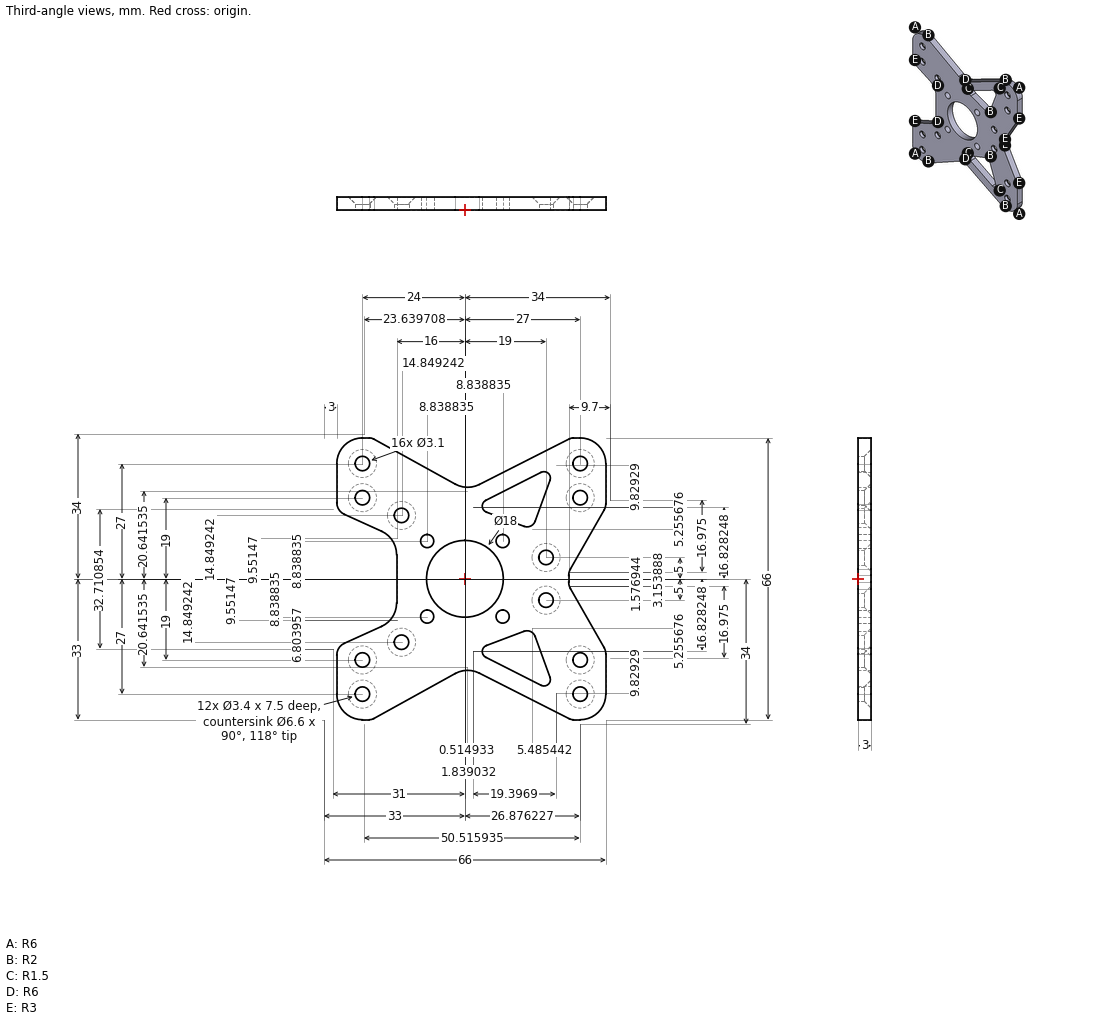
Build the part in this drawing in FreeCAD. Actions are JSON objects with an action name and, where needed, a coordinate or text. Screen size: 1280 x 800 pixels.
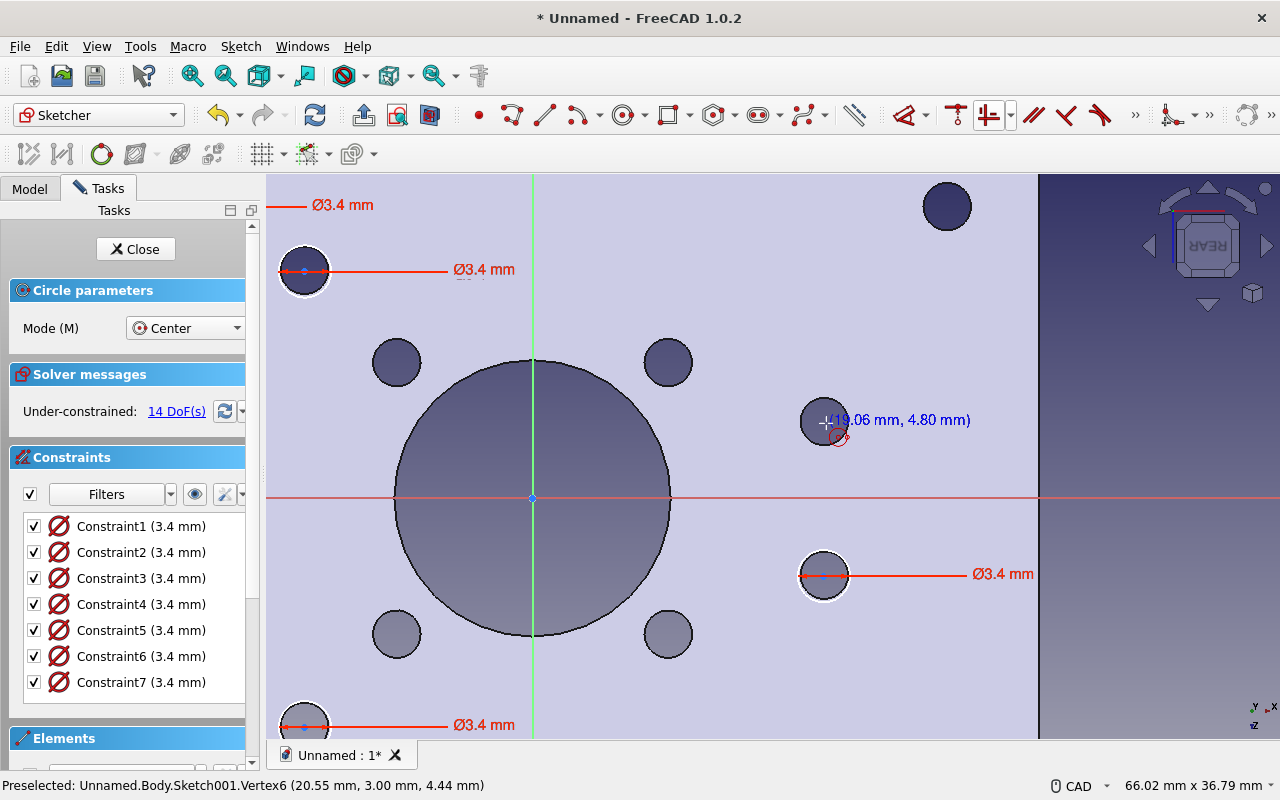
{"action": "left_click", "coordinate": [824, 422]}
{"action": "mouse_move", "coordinate": [843, 403]}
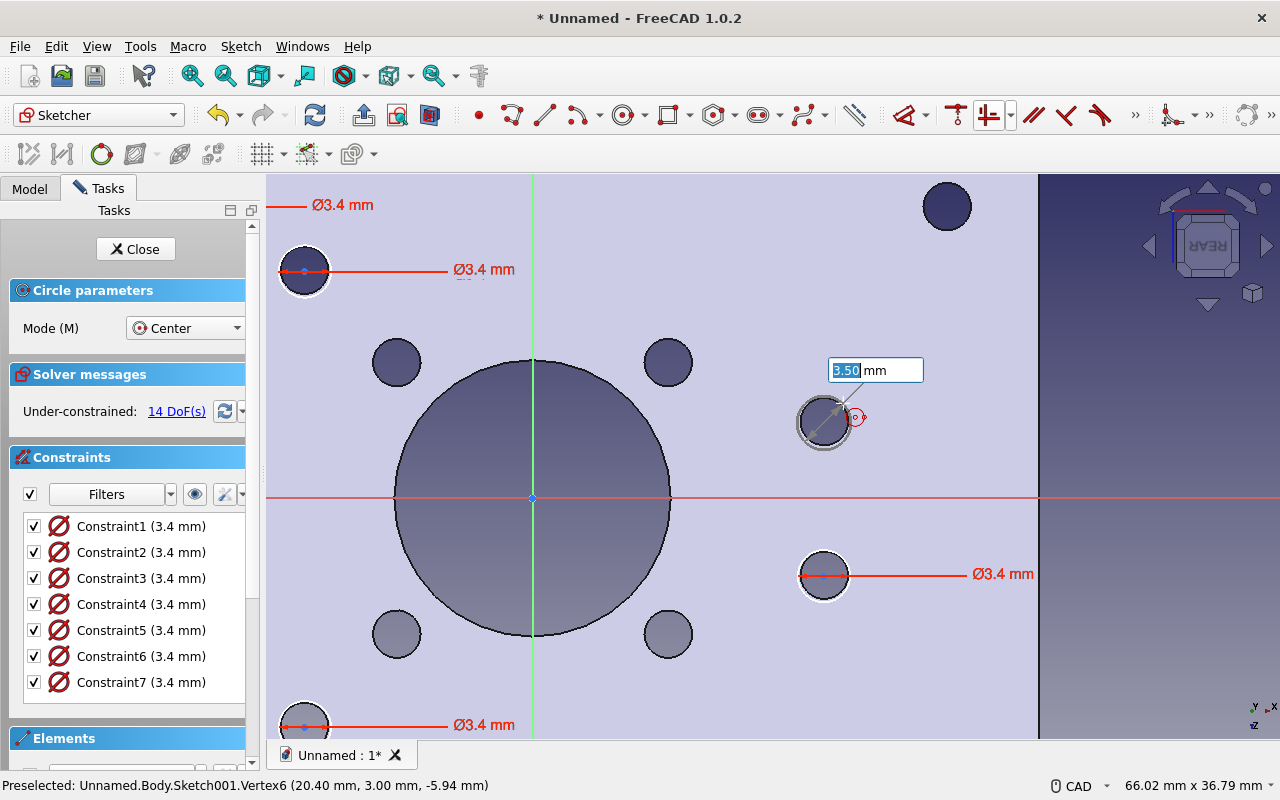
{"action": "type", "text": "3.4"}
{"action": "key", "text": "Return"}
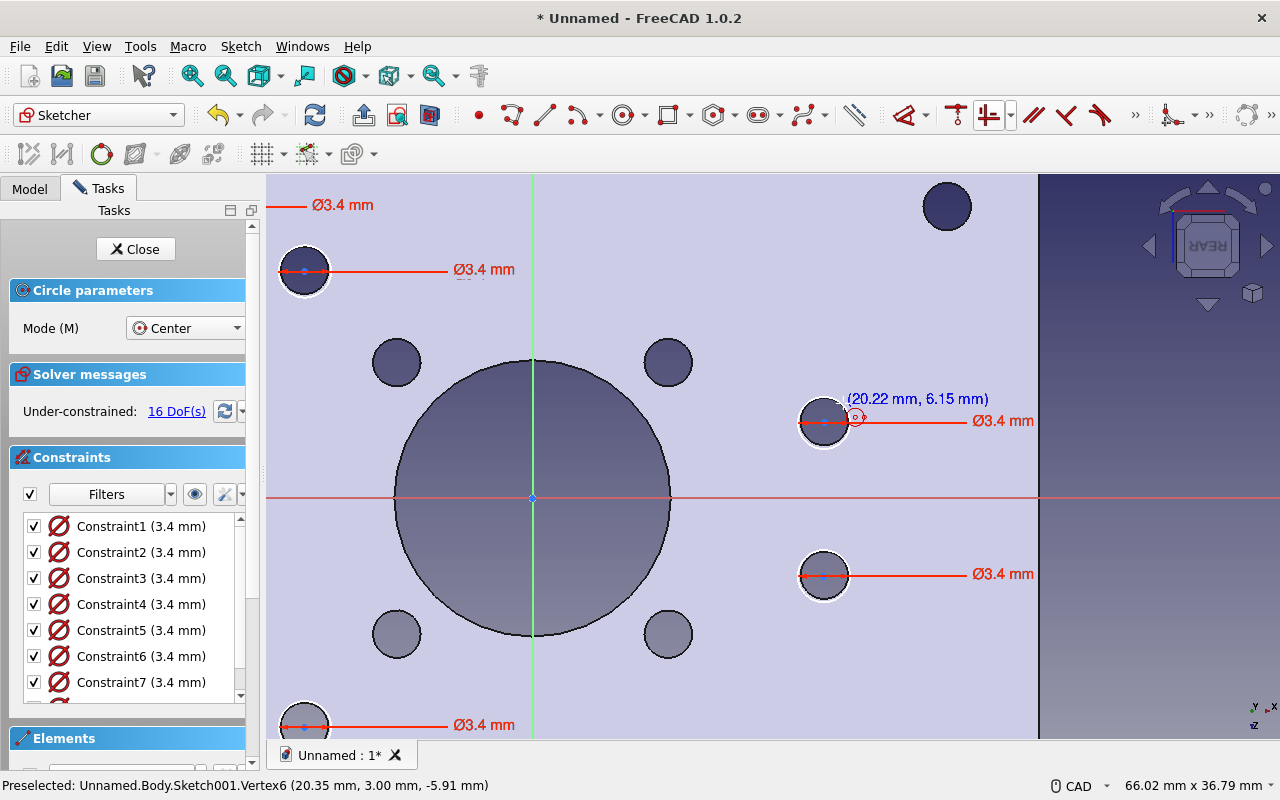
{"action": "left_click", "coordinate": [947, 207]}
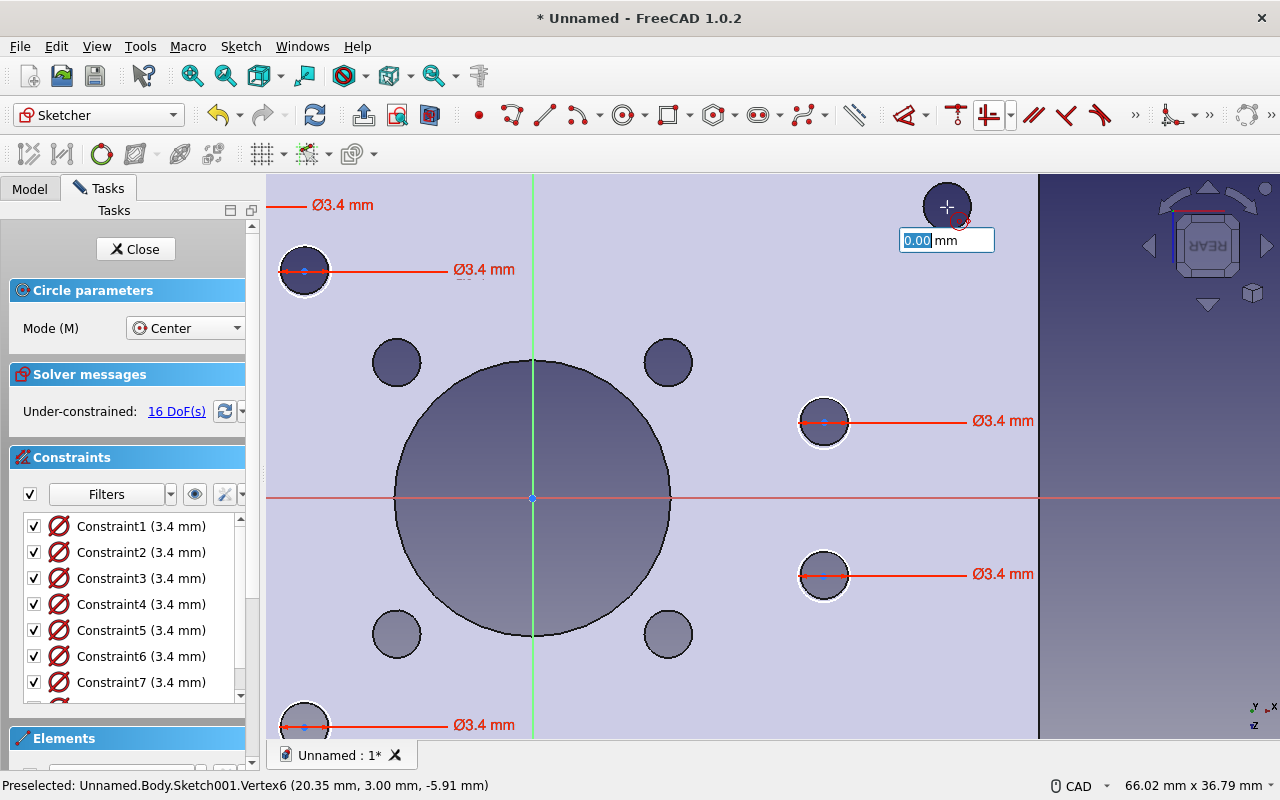
{"action": "scroll", "coordinate": [826, 422], "scroll_direction": "down", "scroll_amount": 4}
{"action": "mouse_move", "coordinate": [889, 317]}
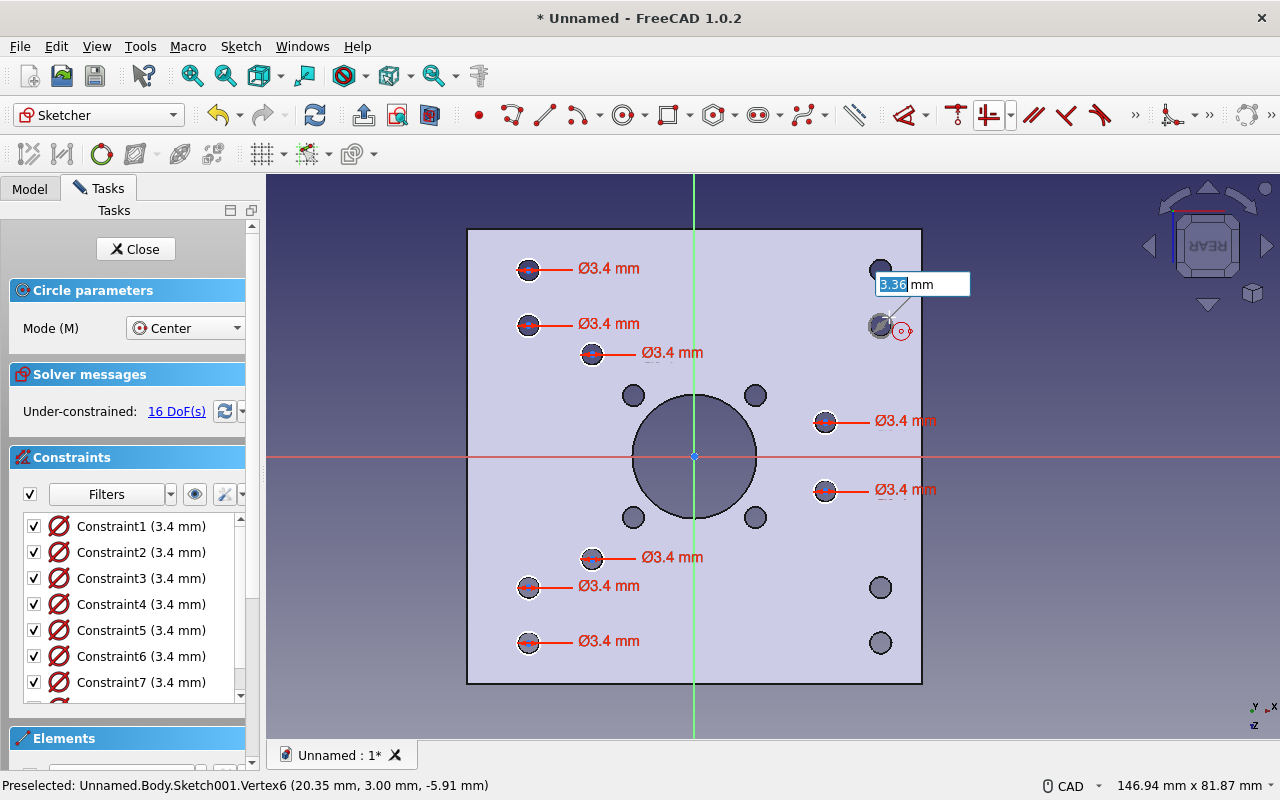
{"action": "type", "text": "3.4"}
{"action": "key", "text": "Return"}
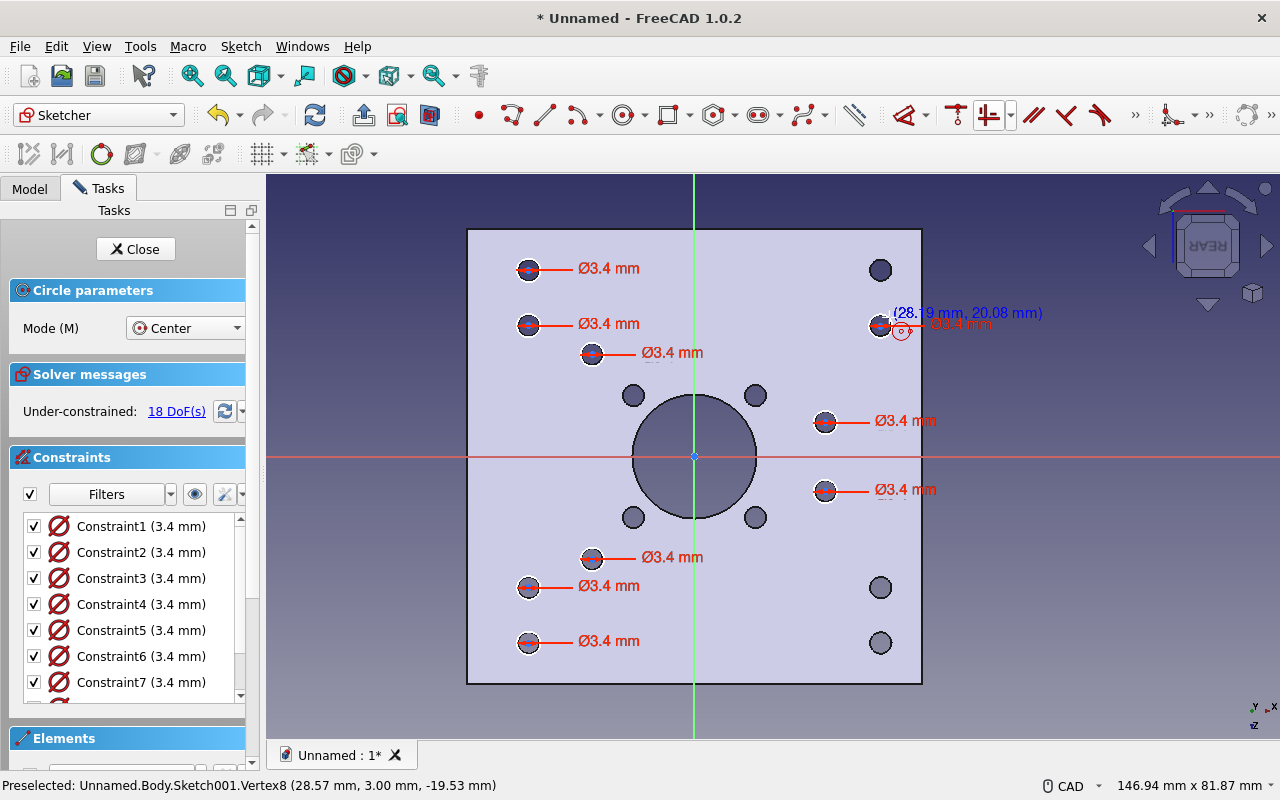
{"action": "scroll", "coordinate": [881, 270], "scroll_direction": "up", "scroll_amount": 4}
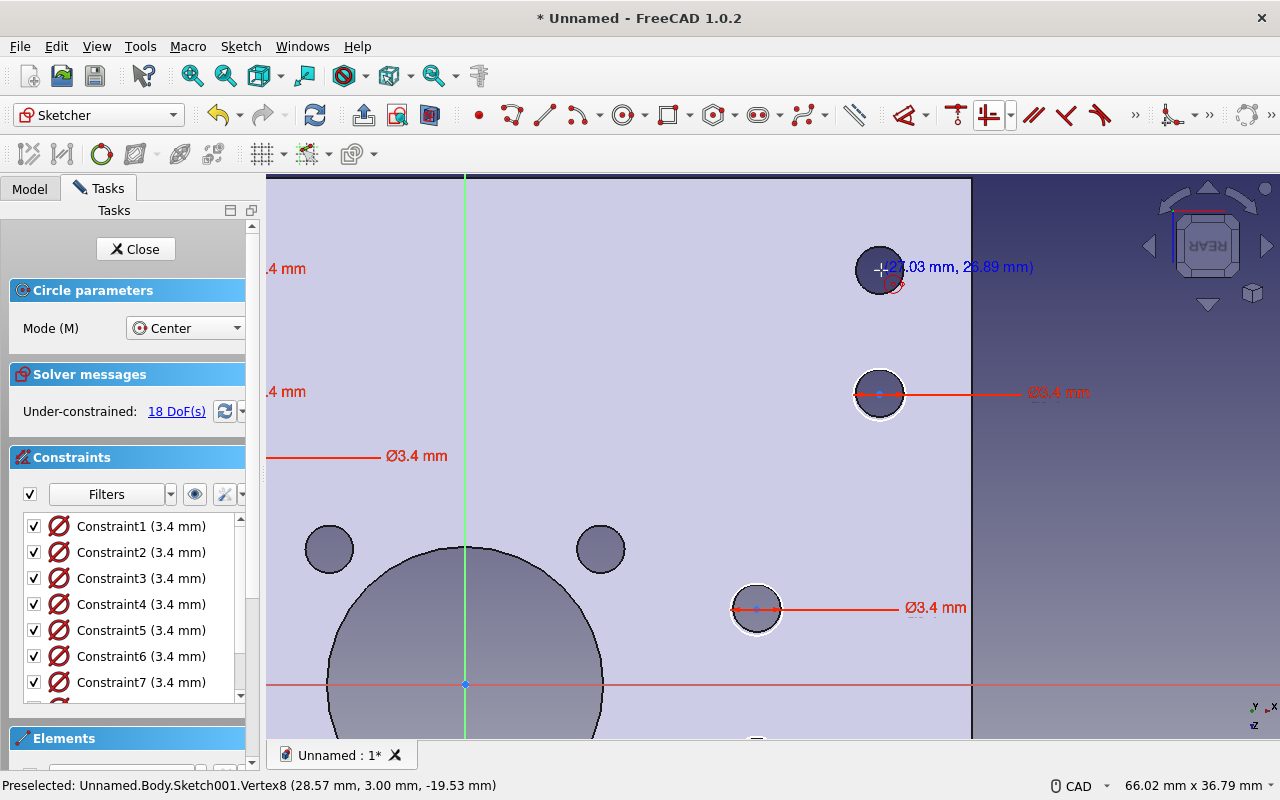
{"action": "left_click", "coordinate": [880, 270]}
{"action": "mouse_move", "coordinate": [898, 252]}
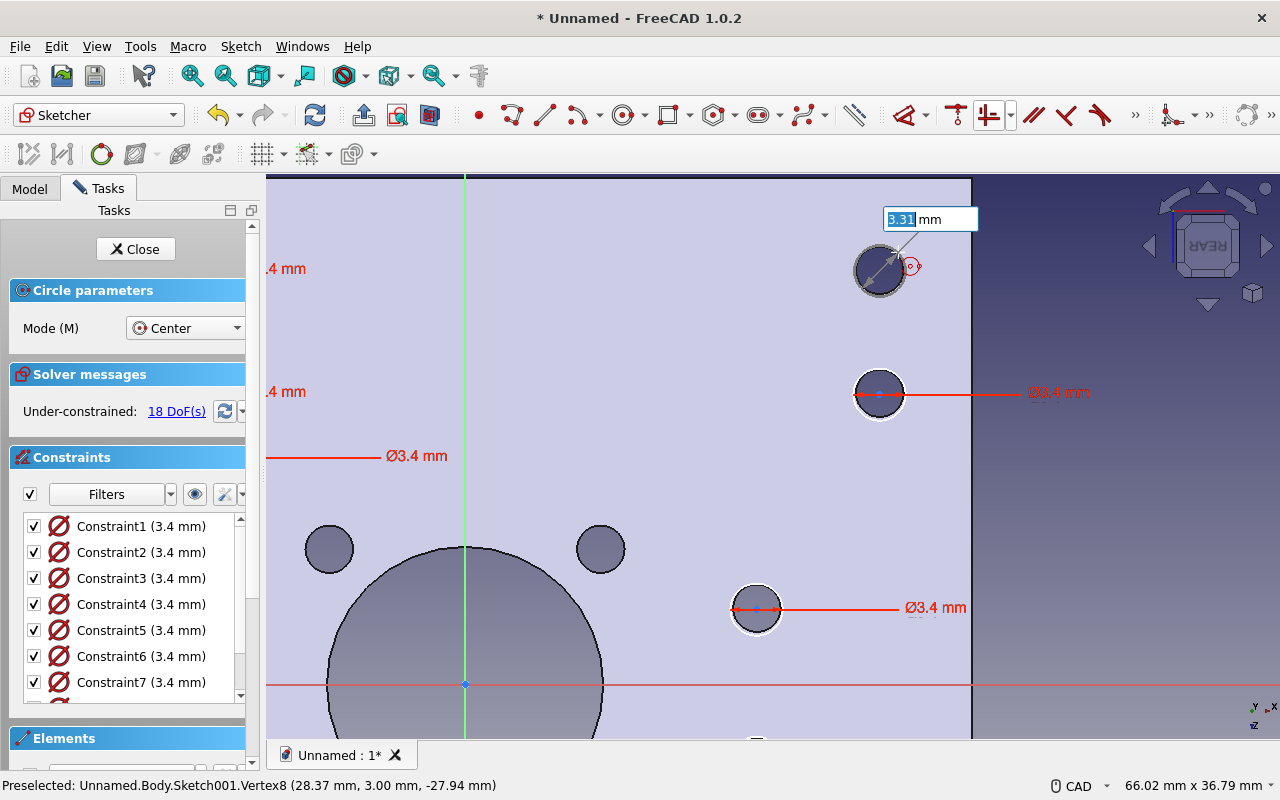
{"action": "type", "text": "3.4"}
{"action": "key", "text": "Return"}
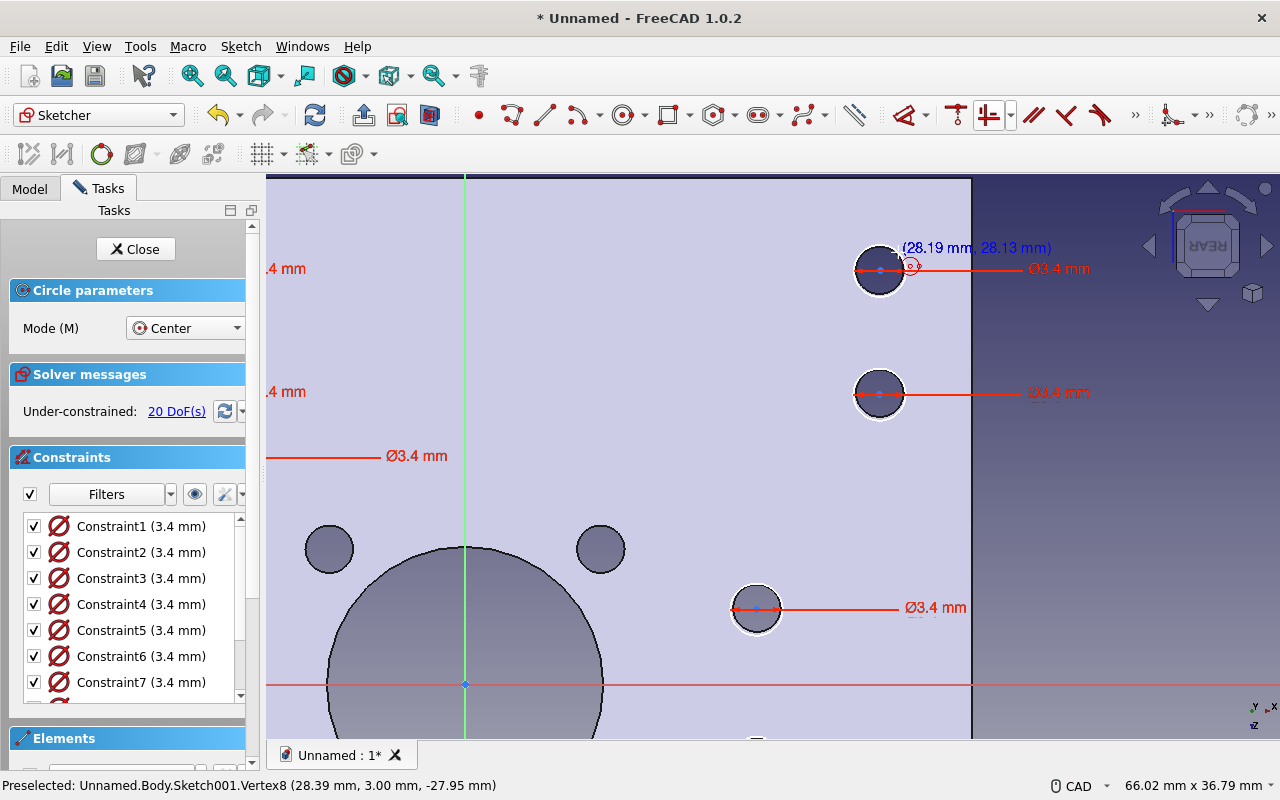
{"action": "scroll", "coordinate": [881, 270], "scroll_direction": "down", "scroll_amount": 4}